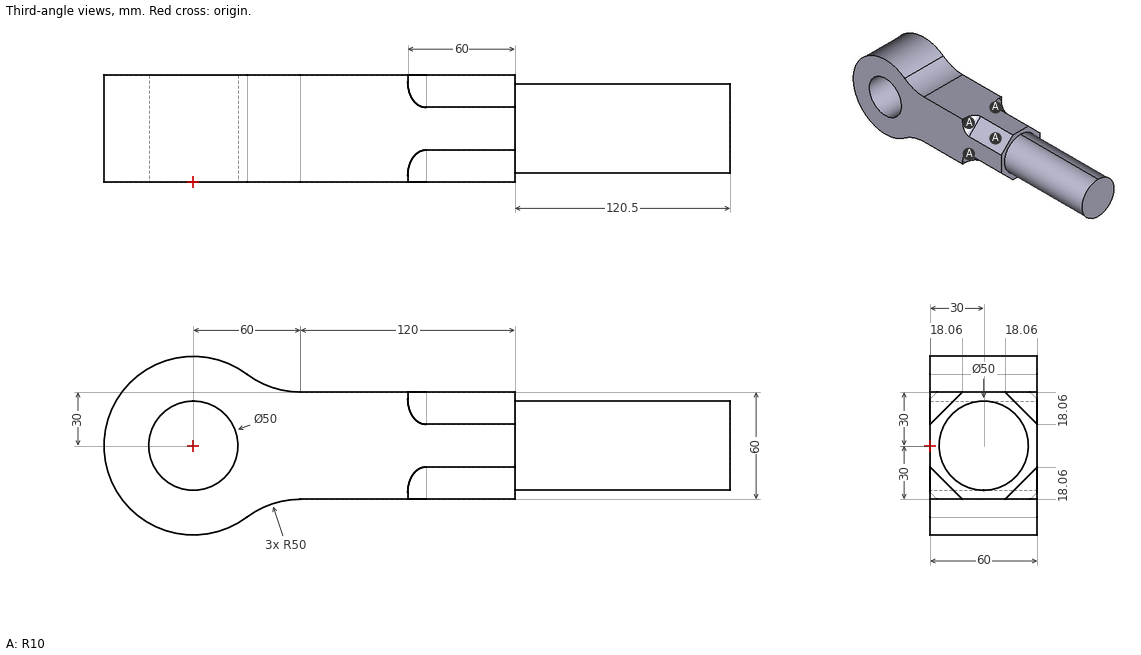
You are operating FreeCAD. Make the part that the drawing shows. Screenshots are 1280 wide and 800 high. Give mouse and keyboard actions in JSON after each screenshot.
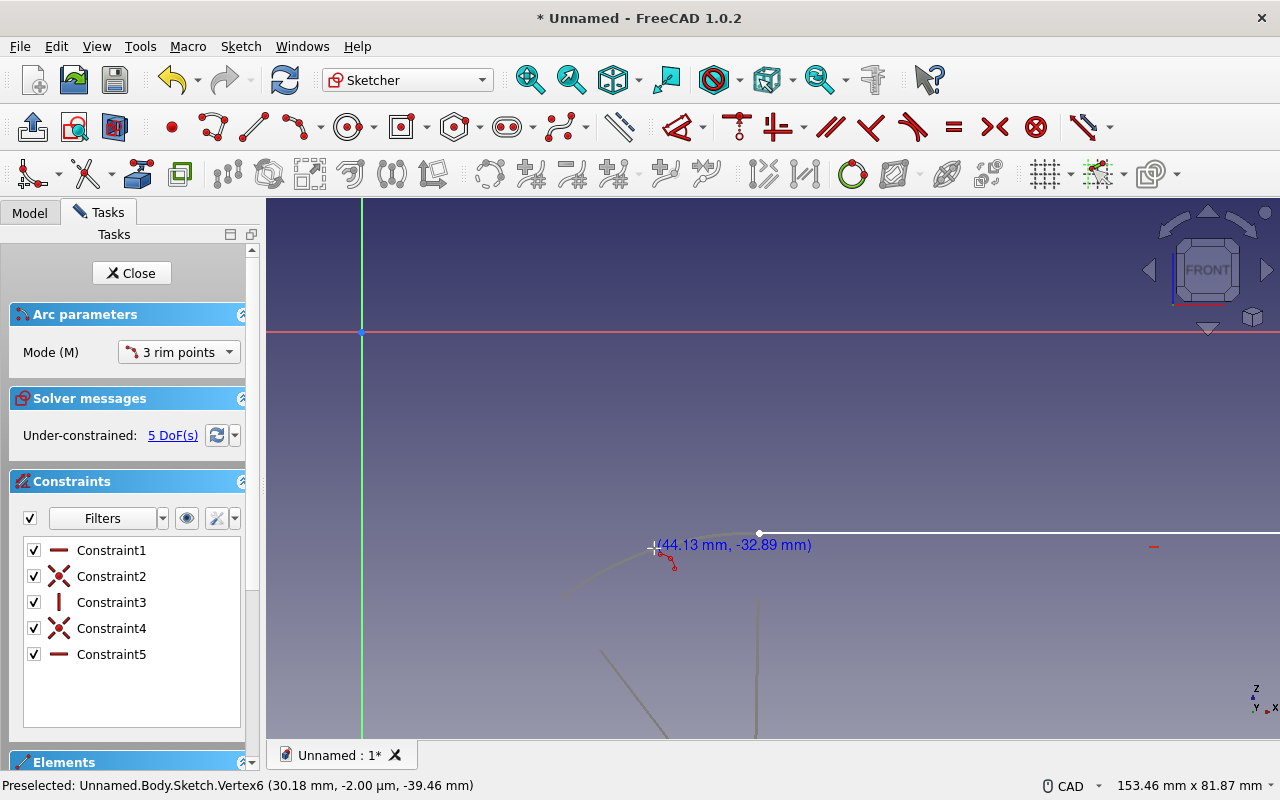
{"action": "left_click", "coordinate": [654, 547]}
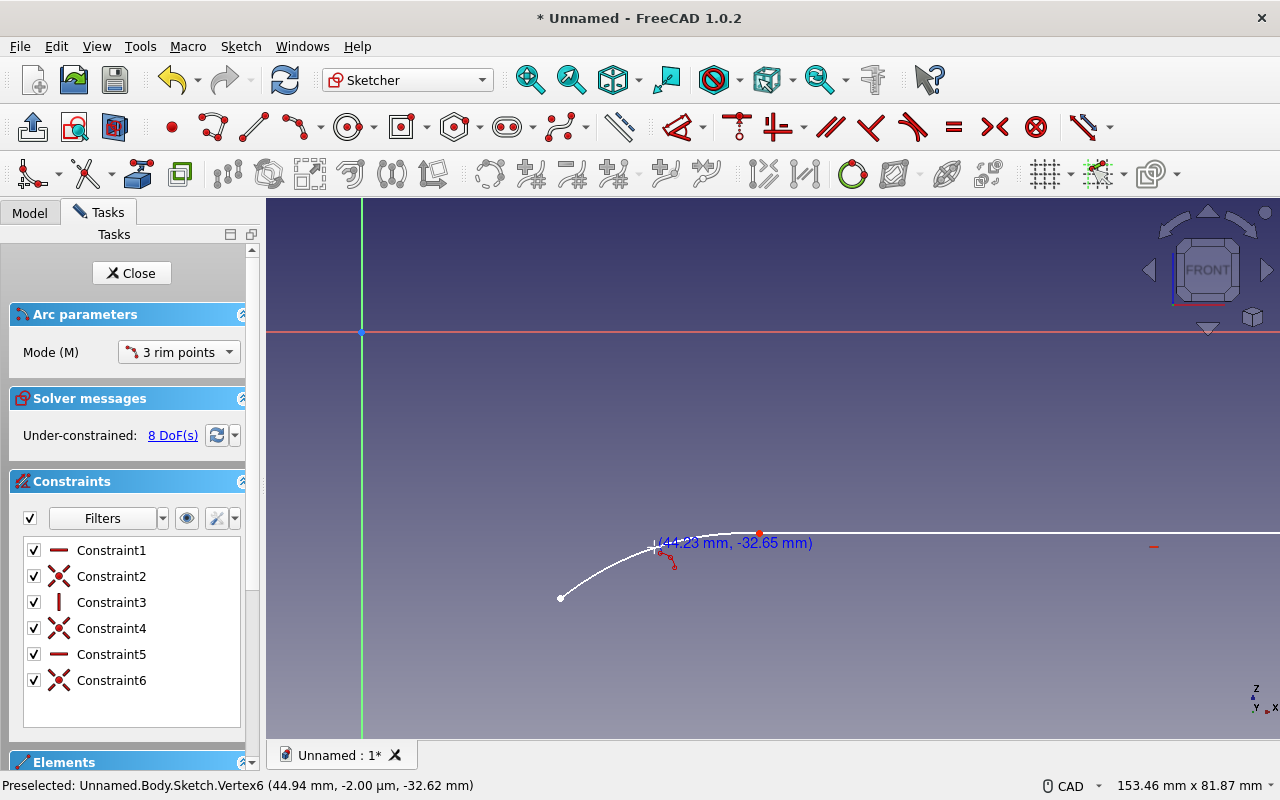
{"action": "left_click", "coordinate": [561, 599]}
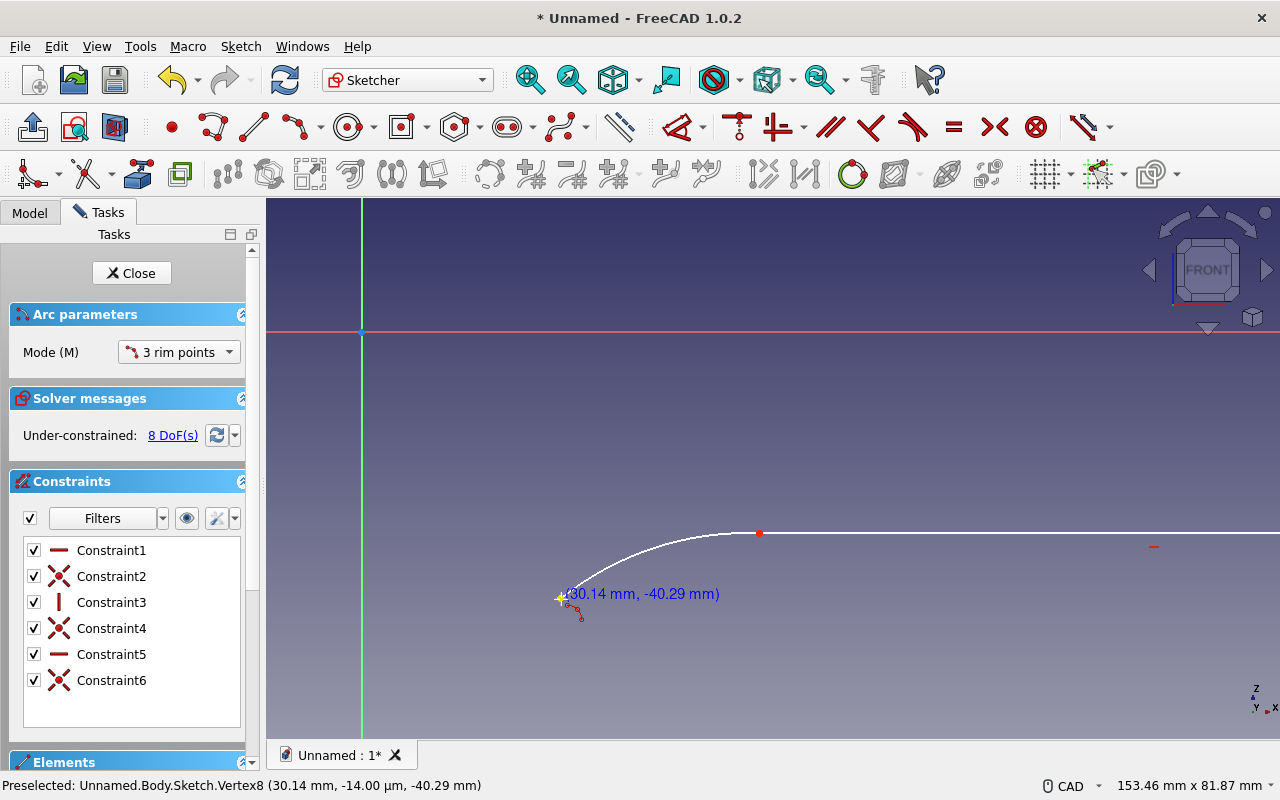
{"action": "scroll", "coordinate": [654, 548], "scroll_direction": "down", "scroll_amount": 5}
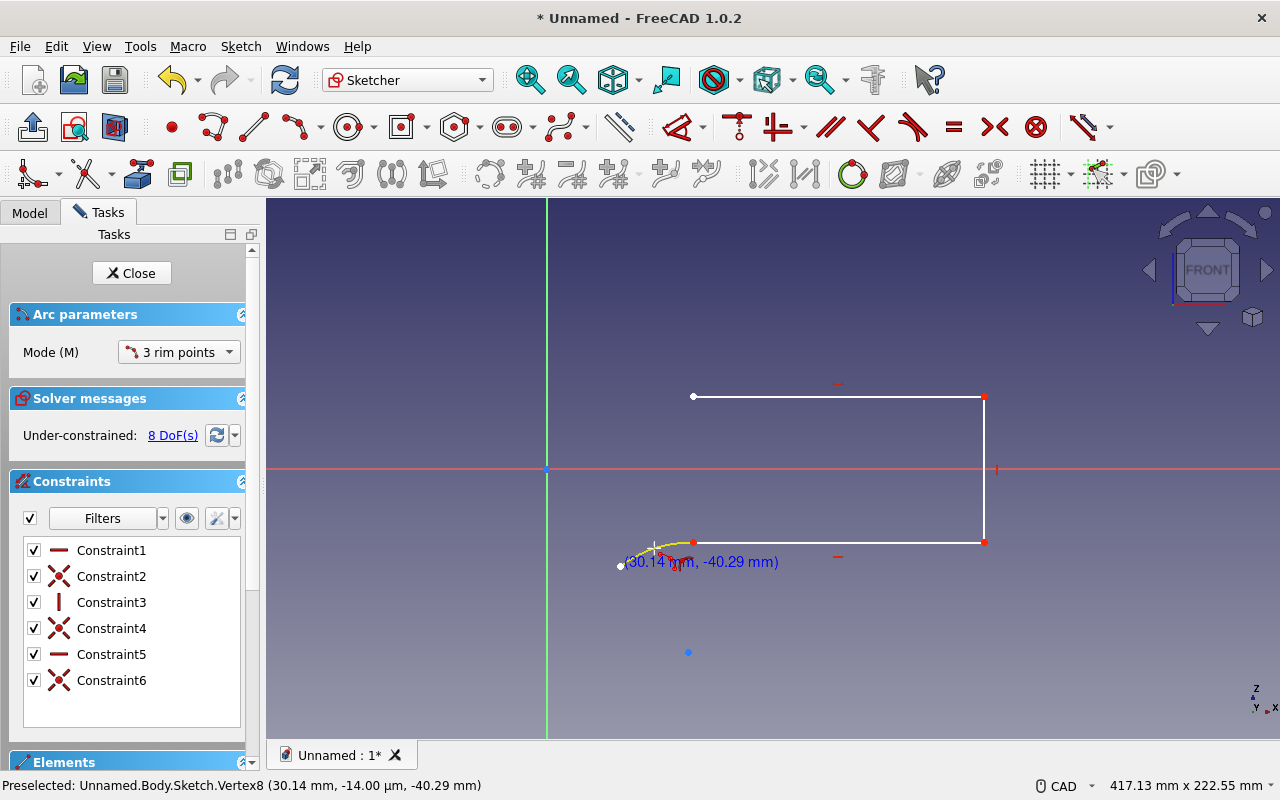
{"action": "left_click", "coordinate": [620, 372]}
{"action": "left_click", "coordinate": [437, 417]}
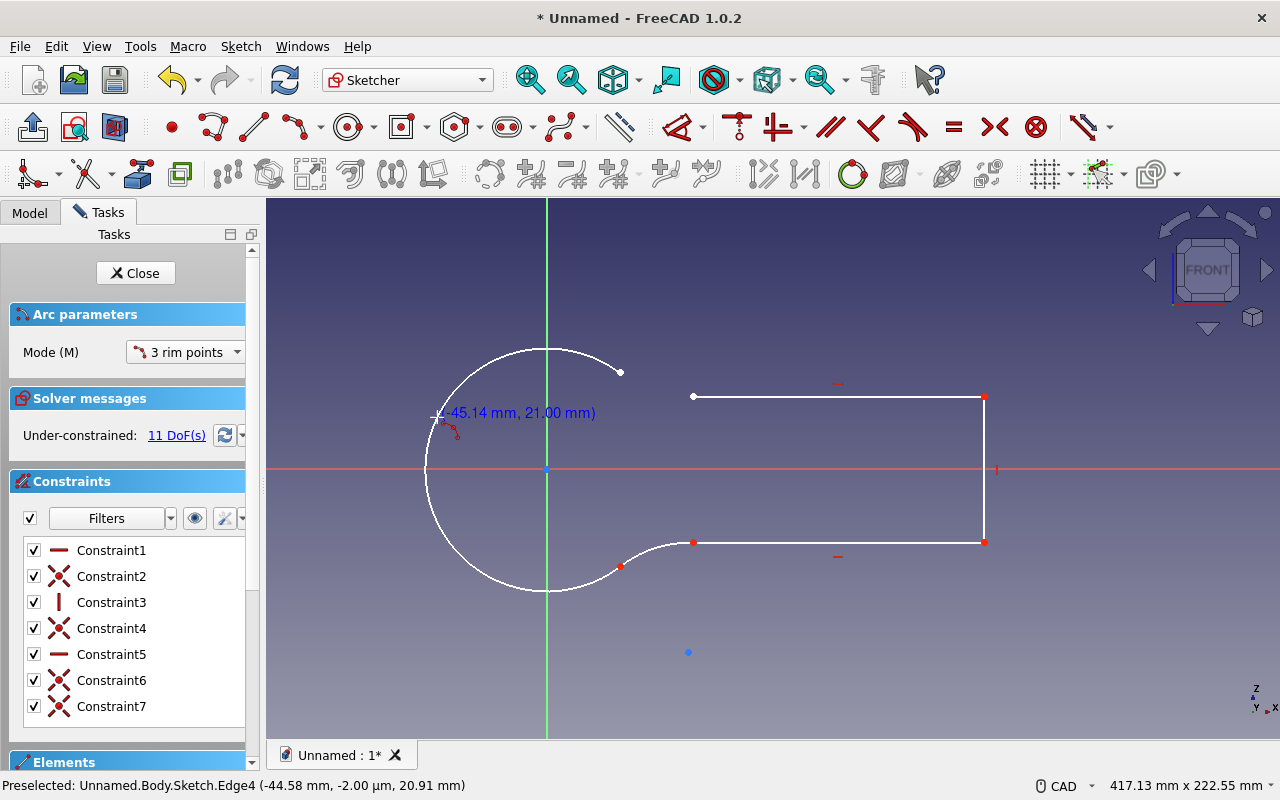
{"action": "left_click", "coordinate": [620, 373]}
{"action": "left_click", "coordinate": [693, 397]}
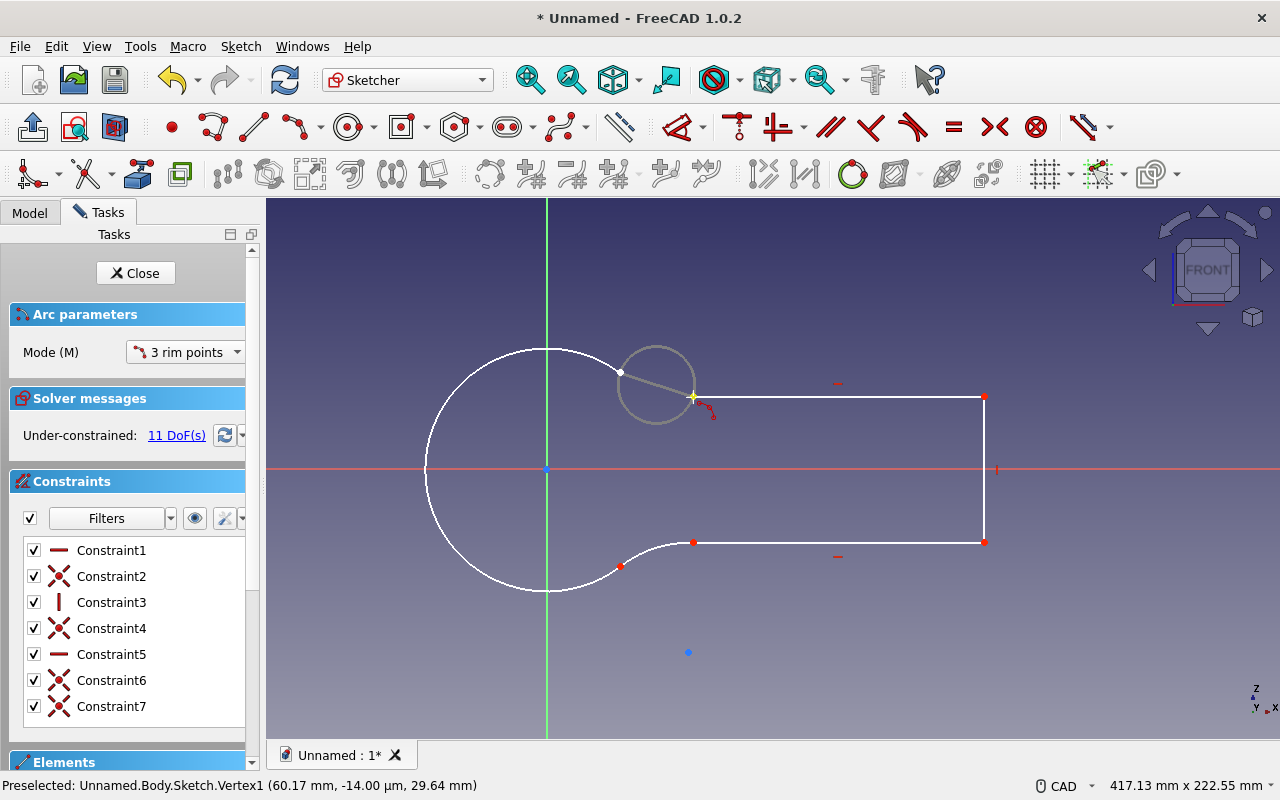
{"action": "scroll", "coordinate": [654, 390], "scroll_direction": "up", "scroll_amount": 5}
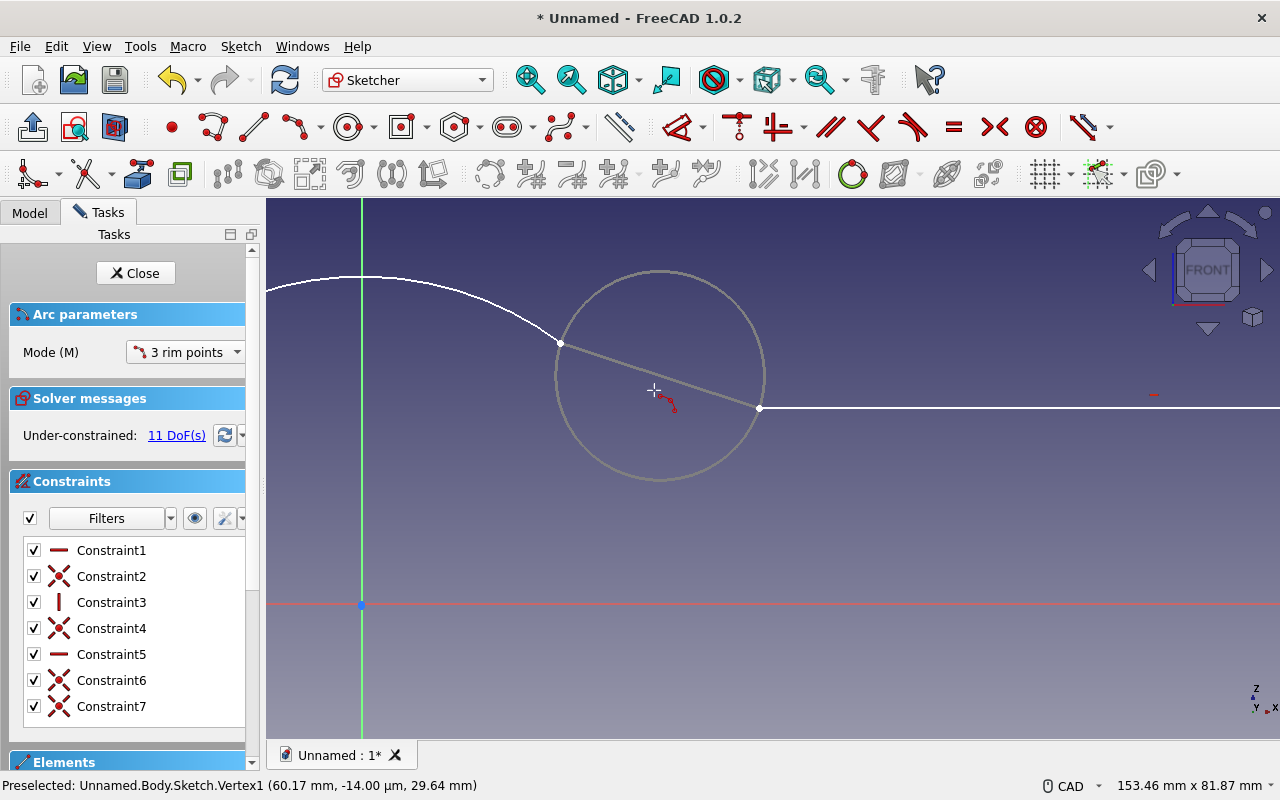
{"action": "left_click", "coordinate": [654, 389]}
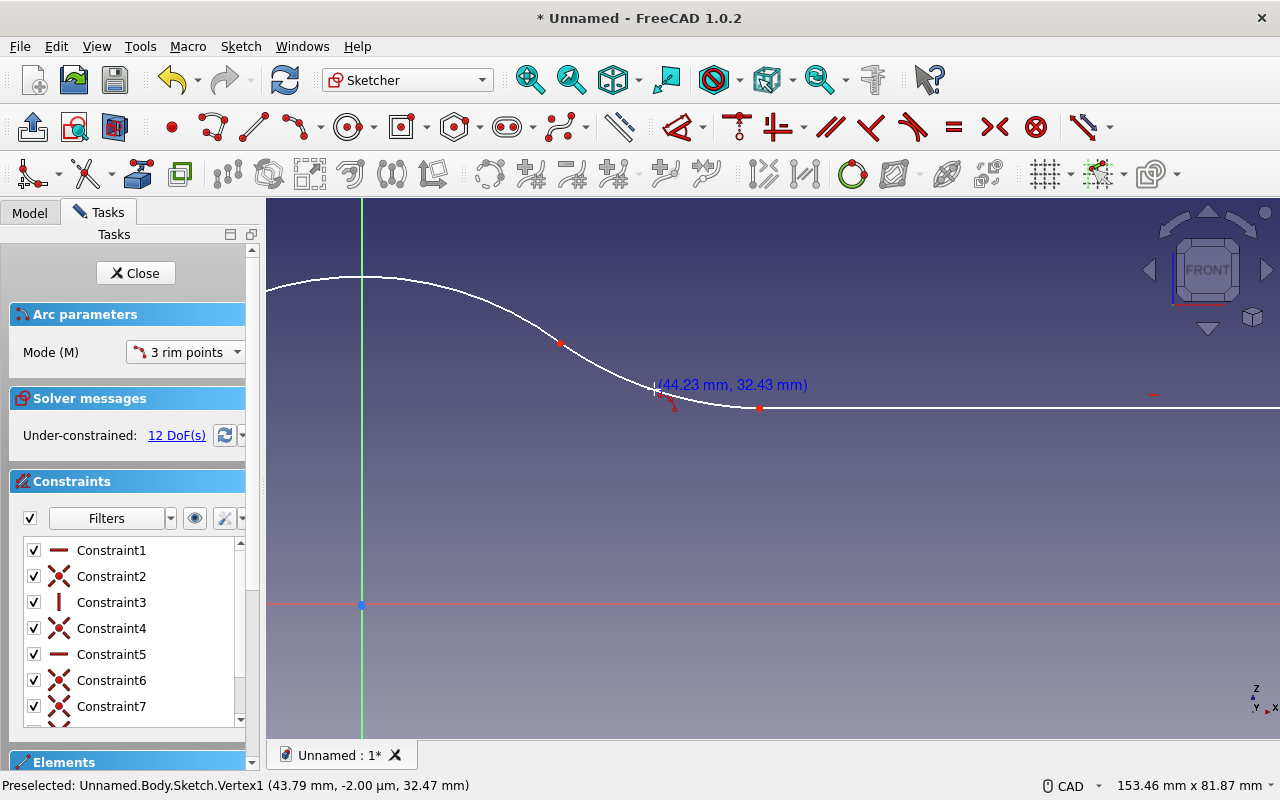
{"action": "key", "text": "g c"}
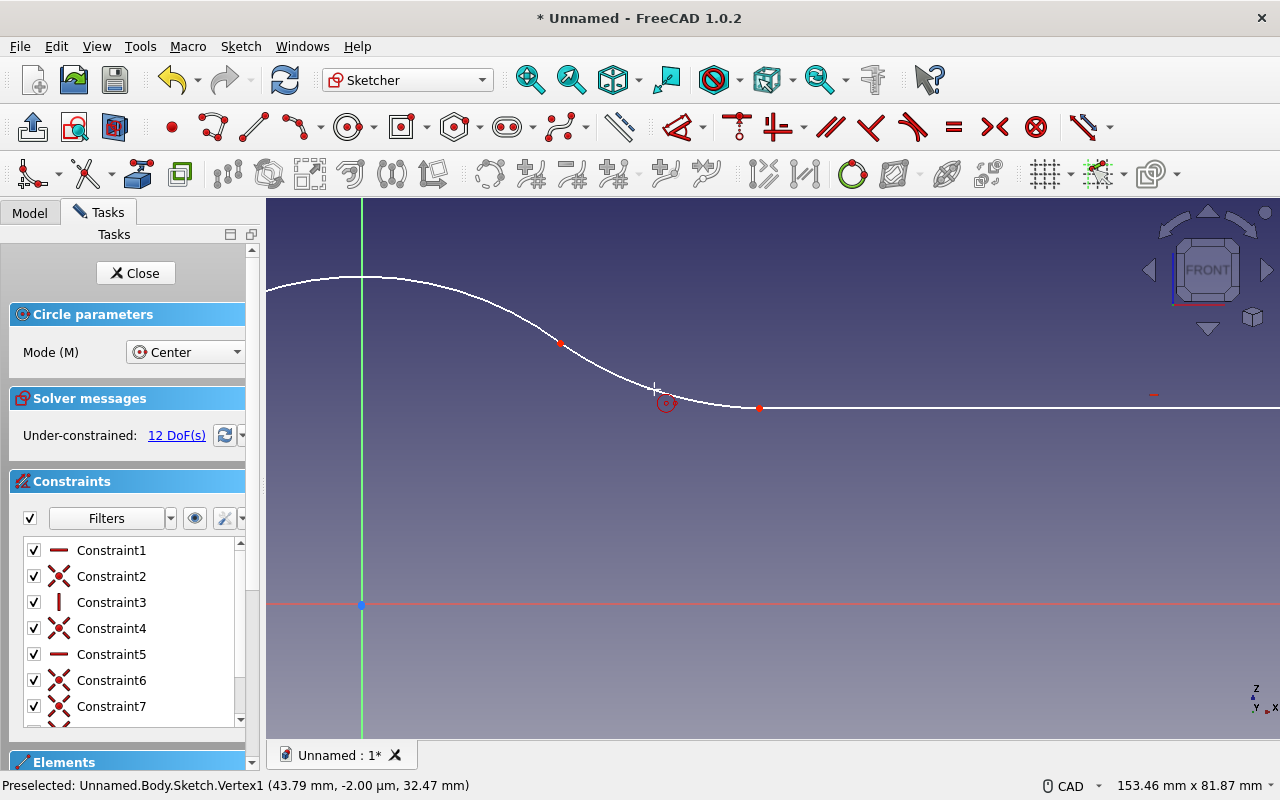
{"action": "left_click", "coordinate": [362, 604]}
{"action": "mouse_move", "coordinate": [479, 487]}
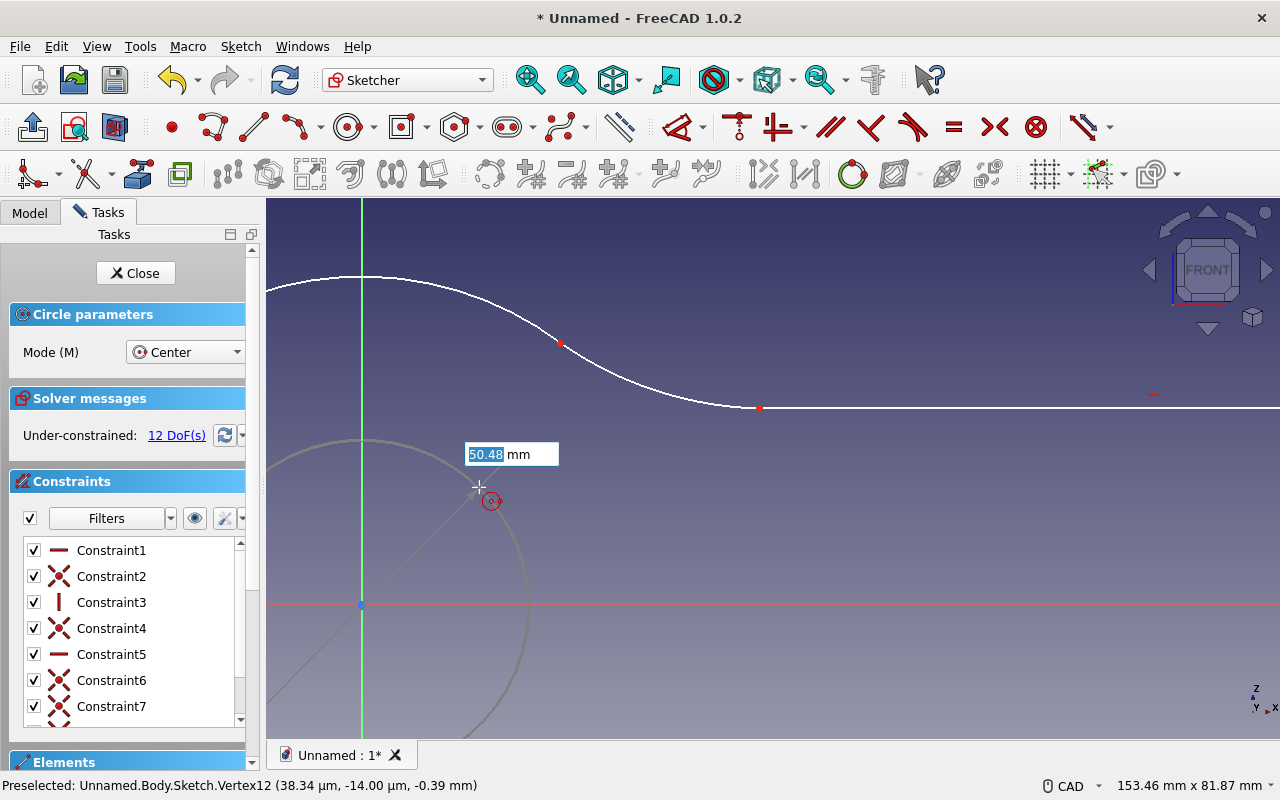
{"action": "type", "text": "50"}
{"action": "key", "text": "Return"}
{"action": "key", "text": "Escape"}